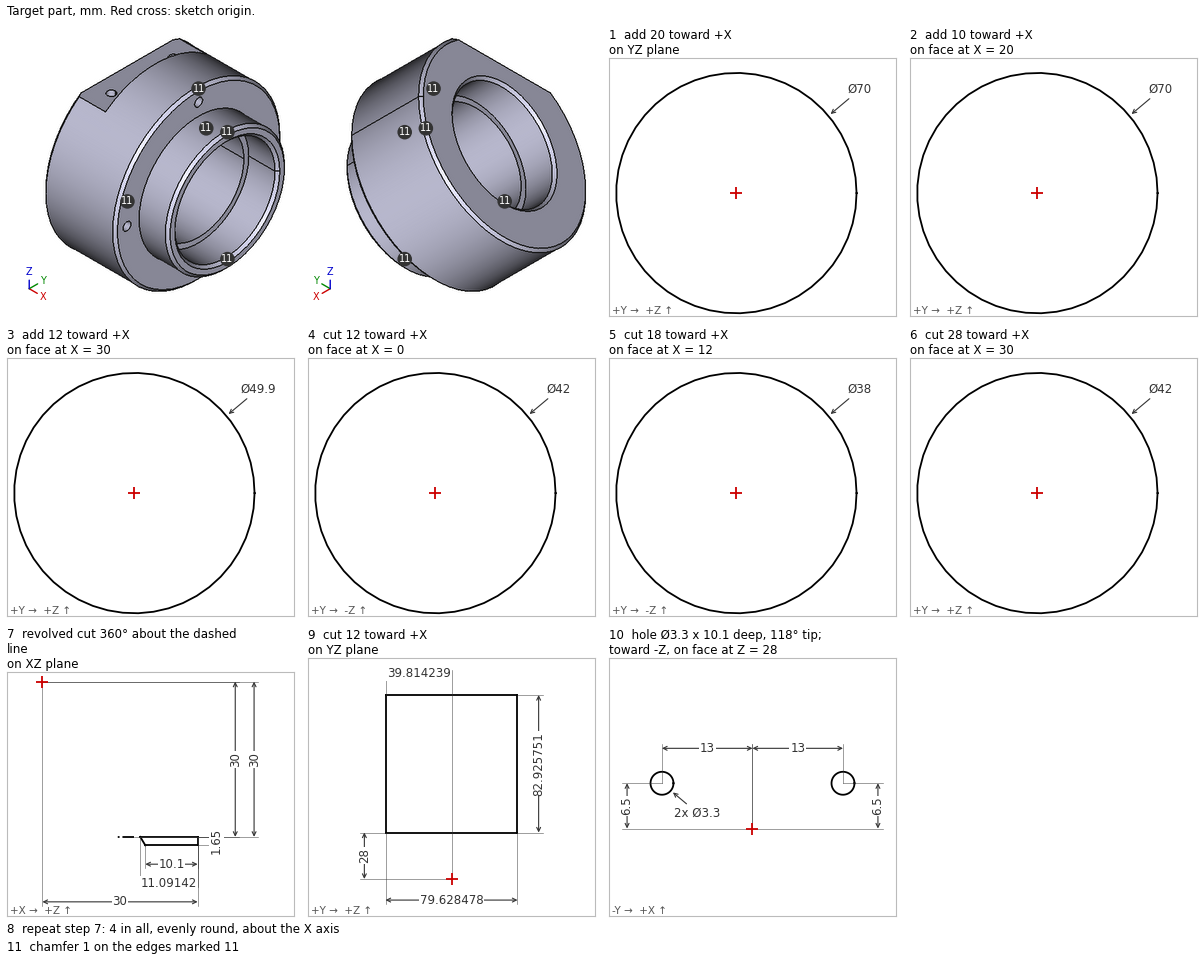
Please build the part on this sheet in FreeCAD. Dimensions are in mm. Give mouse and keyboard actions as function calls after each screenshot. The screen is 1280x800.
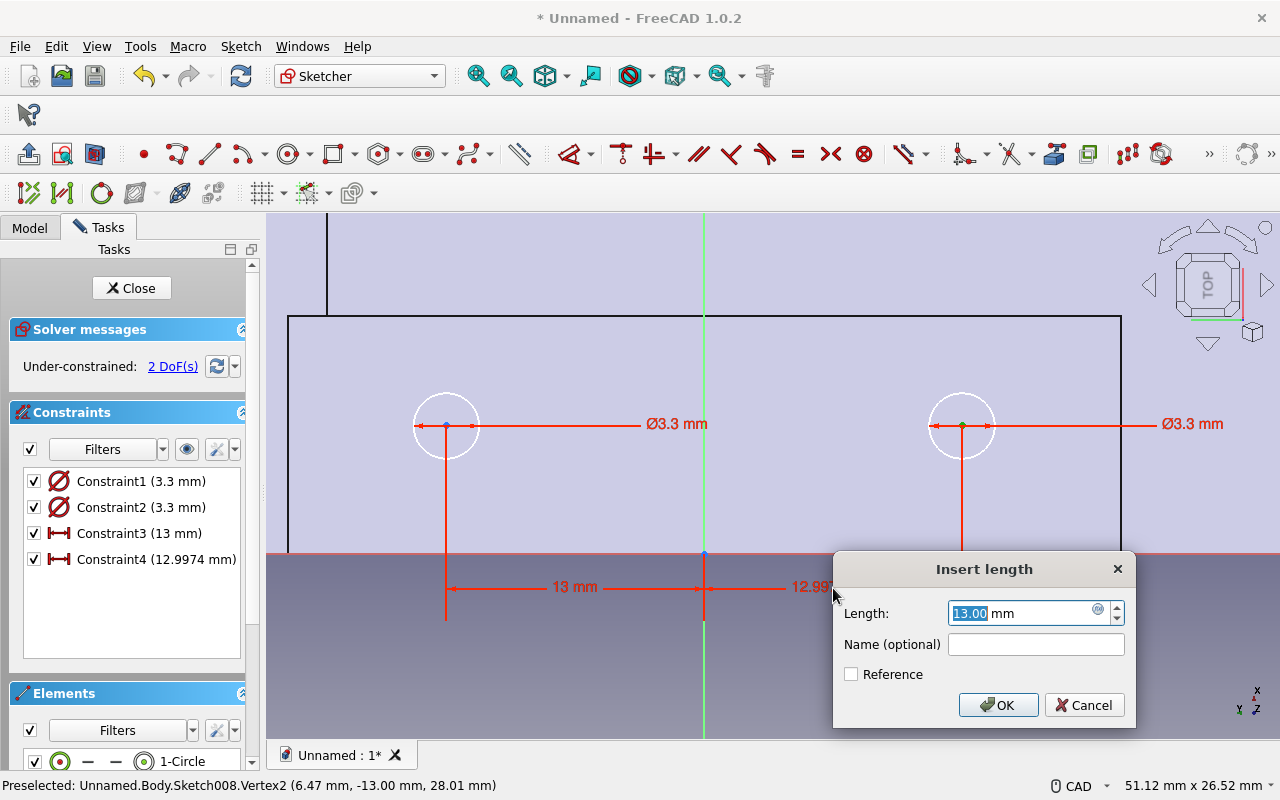
text(13)
key(Return)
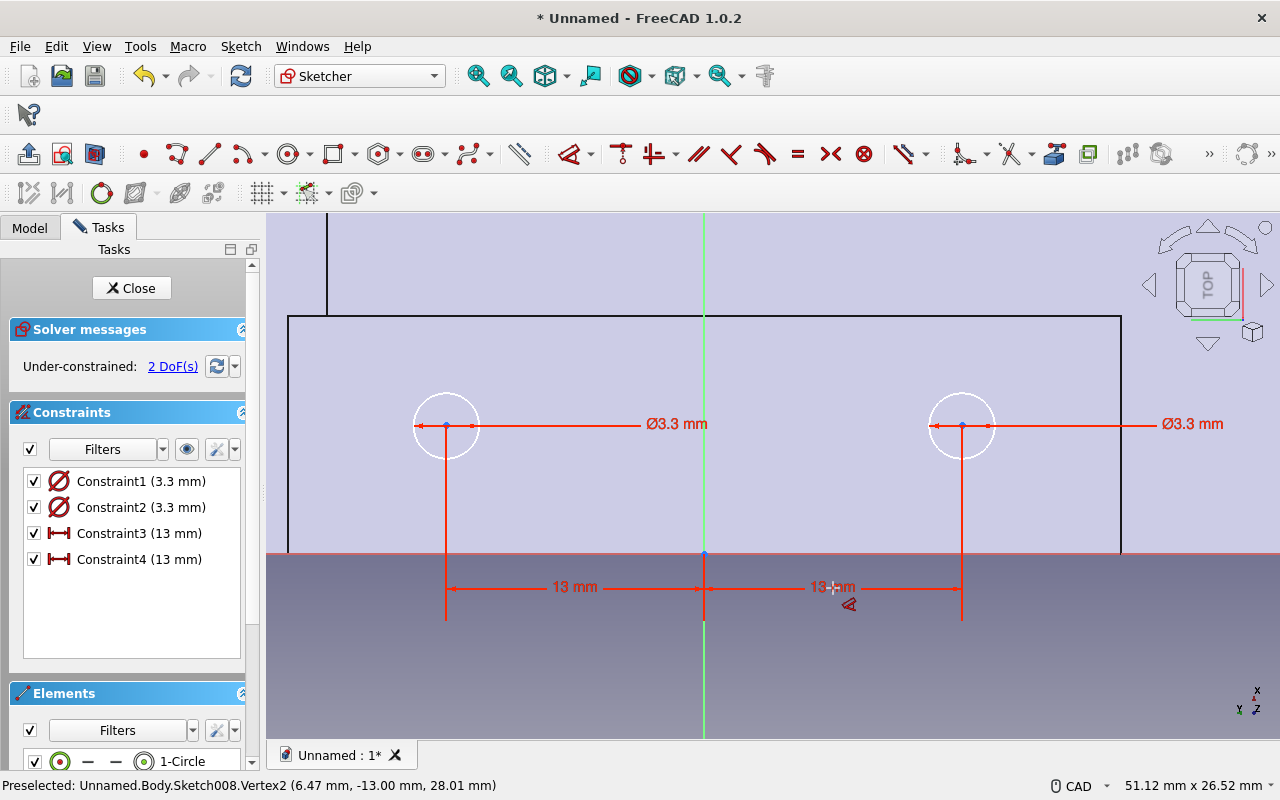
click(446, 426)
click(412, 490)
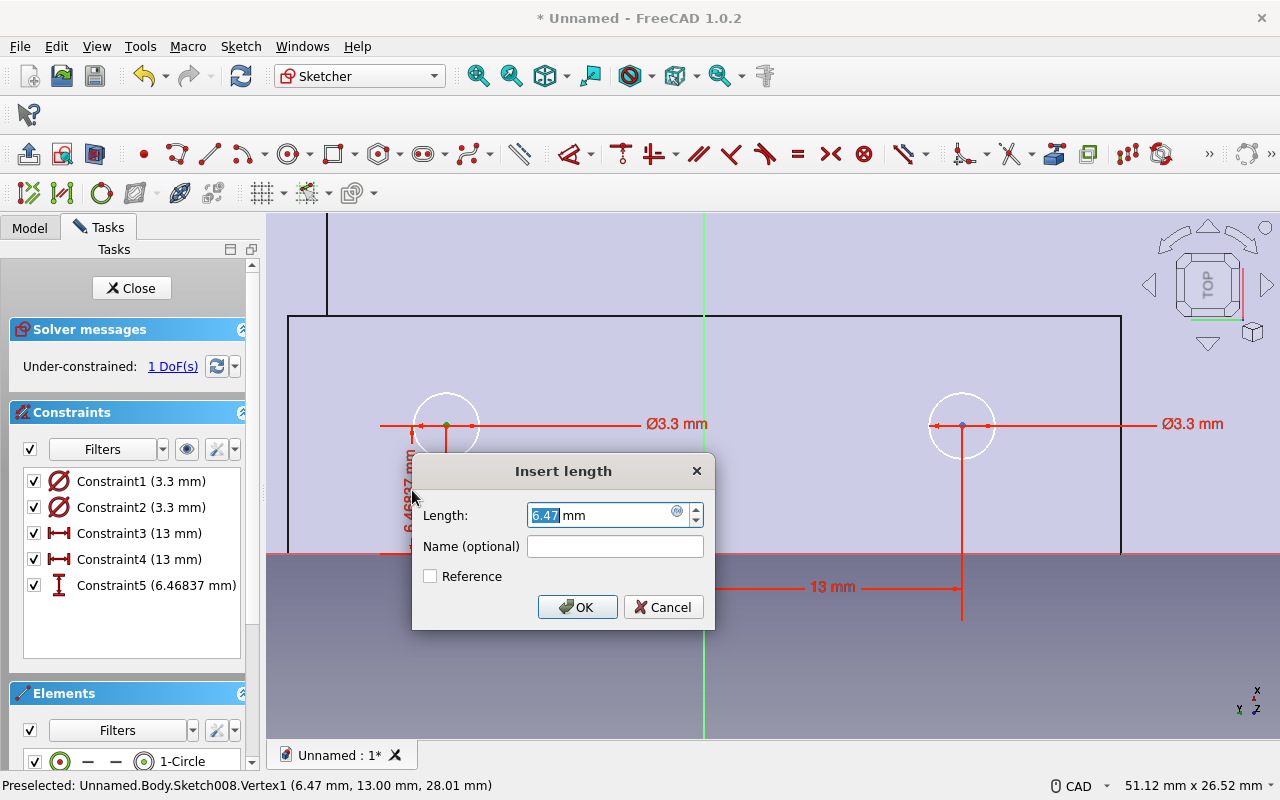
text(6.5)
key(Return)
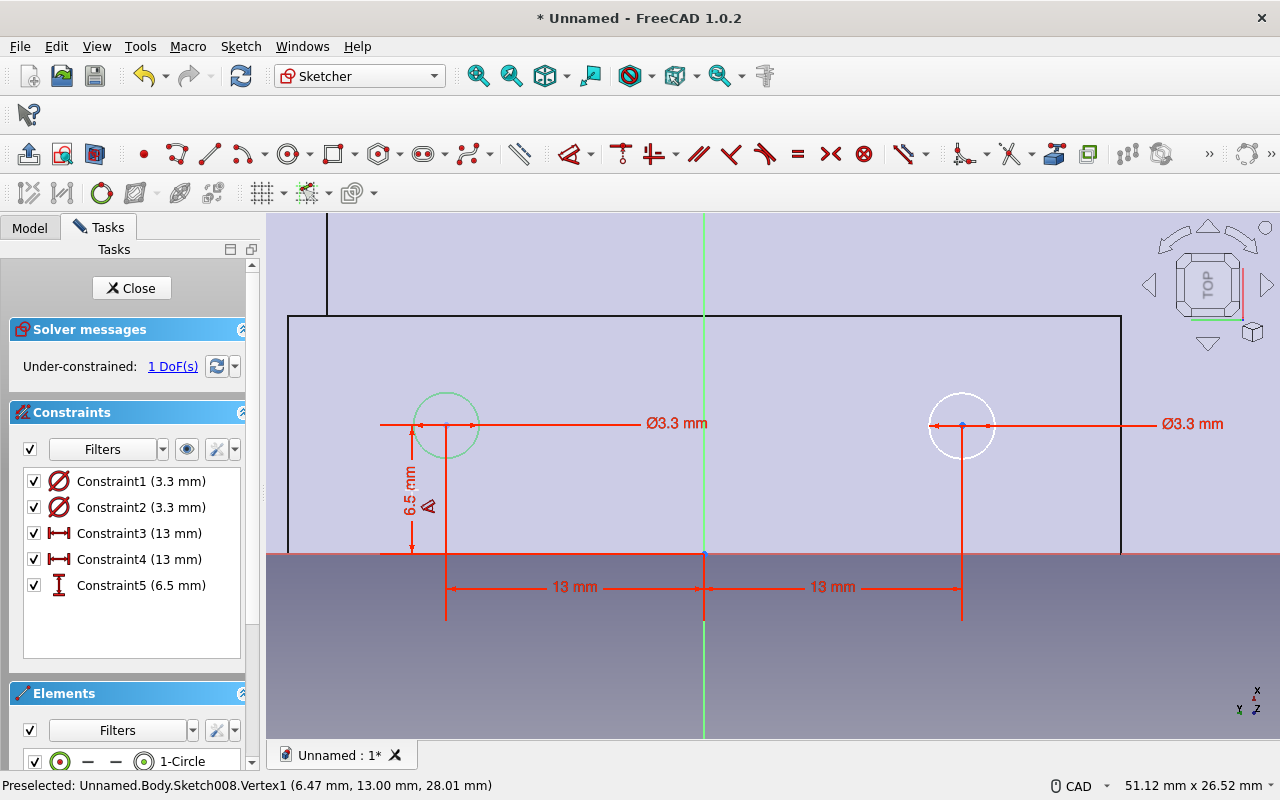
click(962, 426)
click(996, 490)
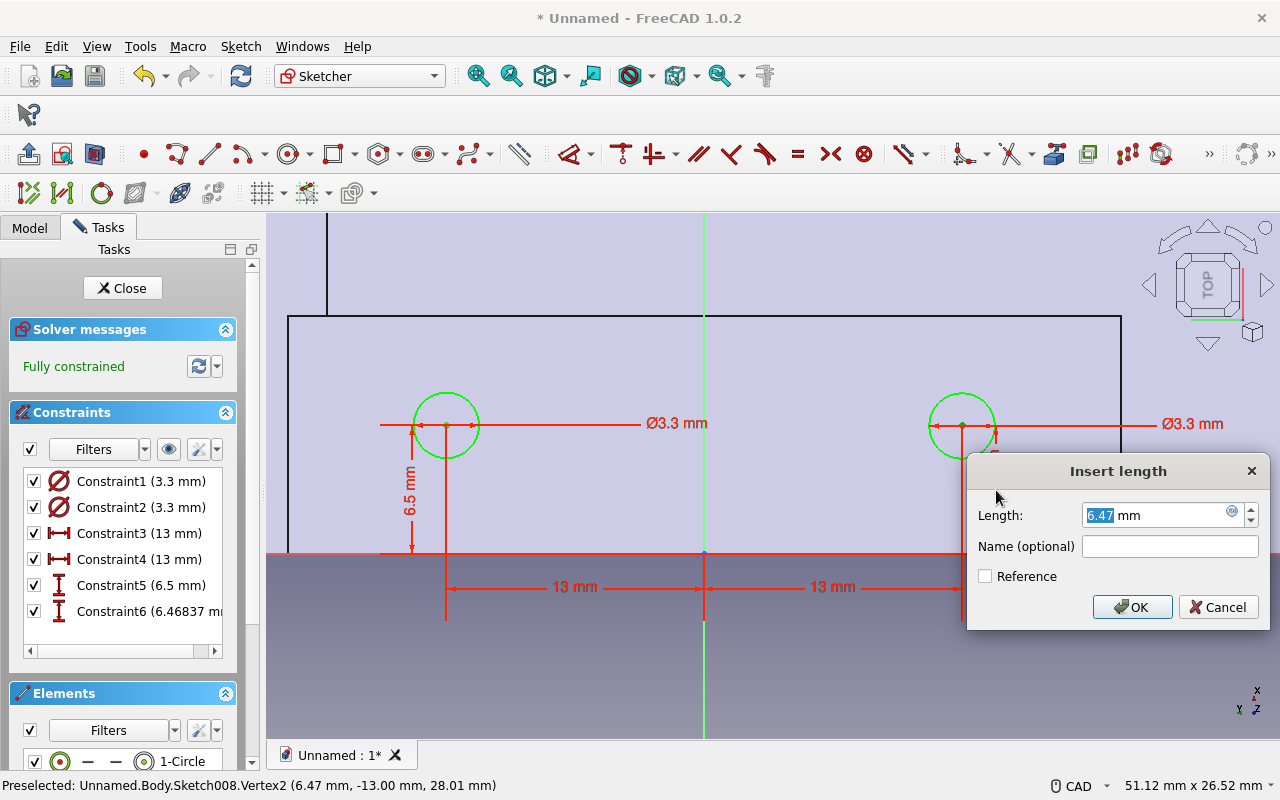
text(6.5)
key(Return)
key(Escape)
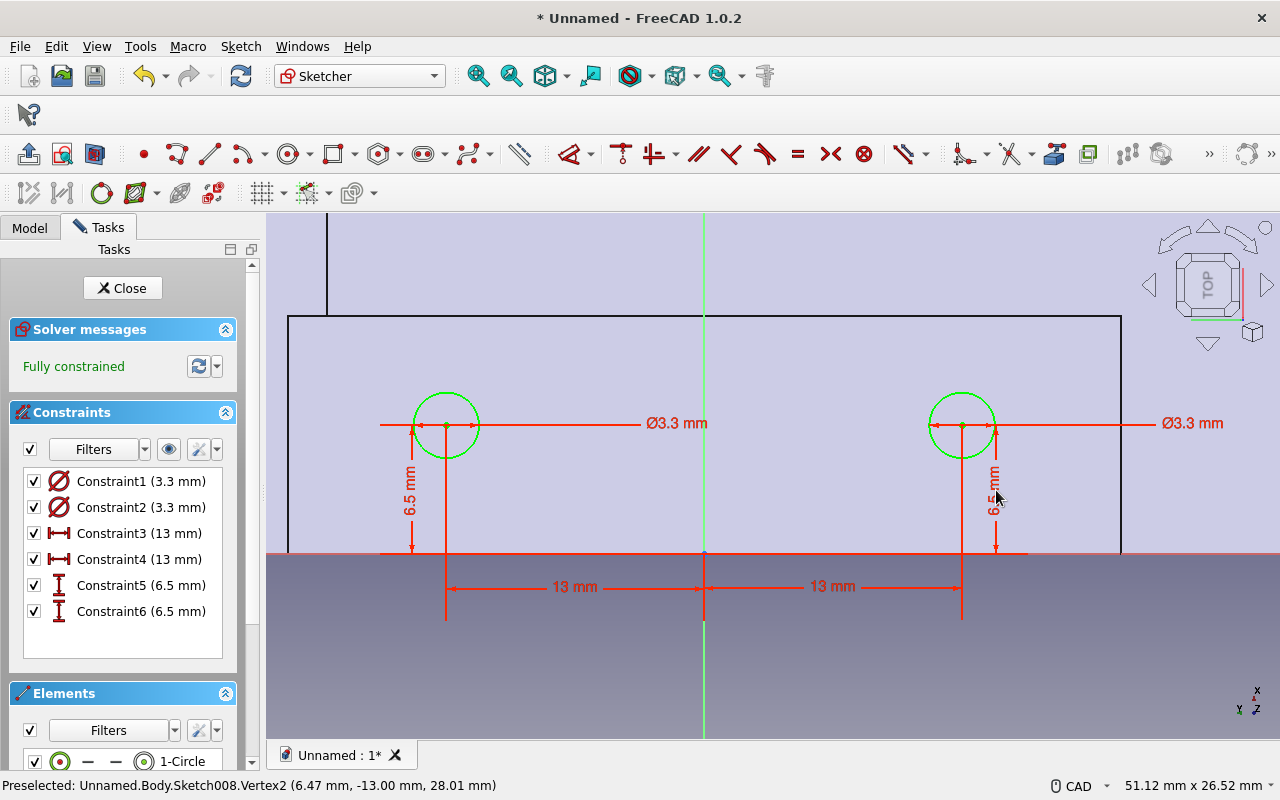
click(123, 288)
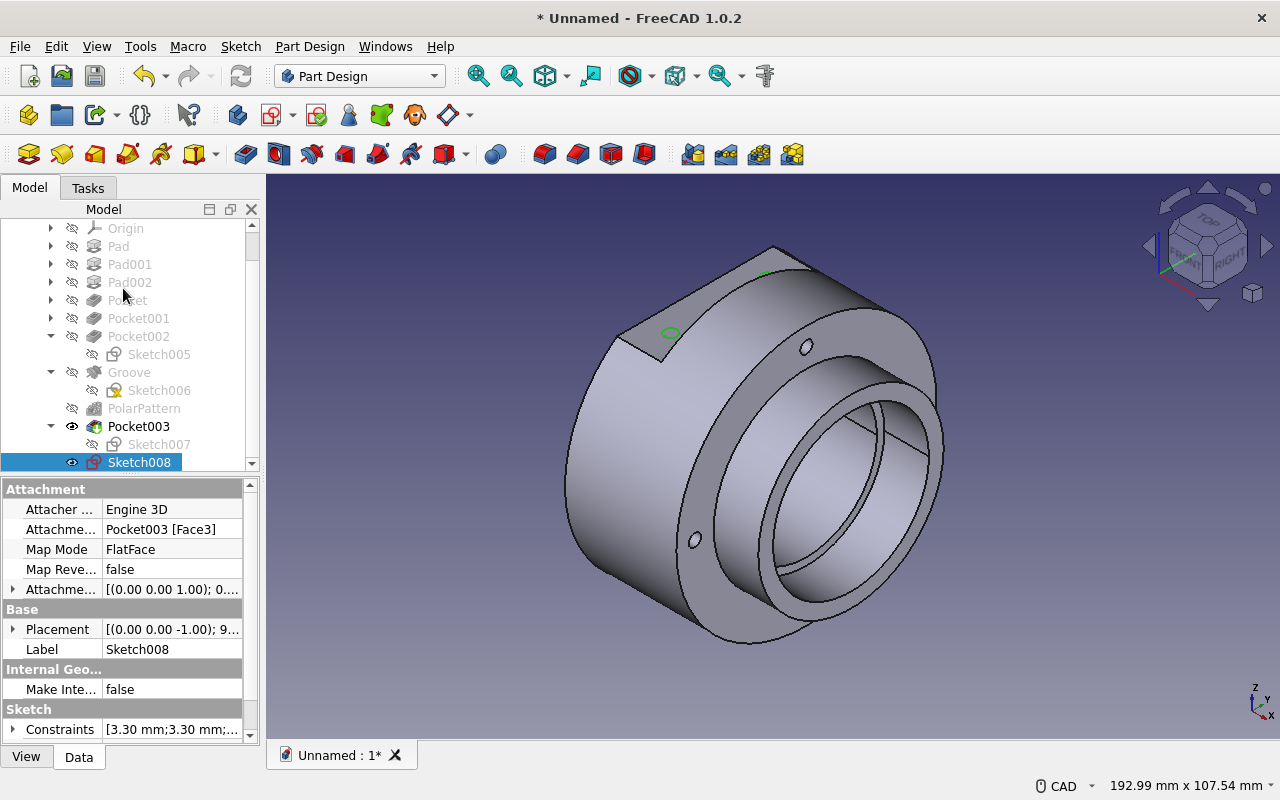
click(279, 154)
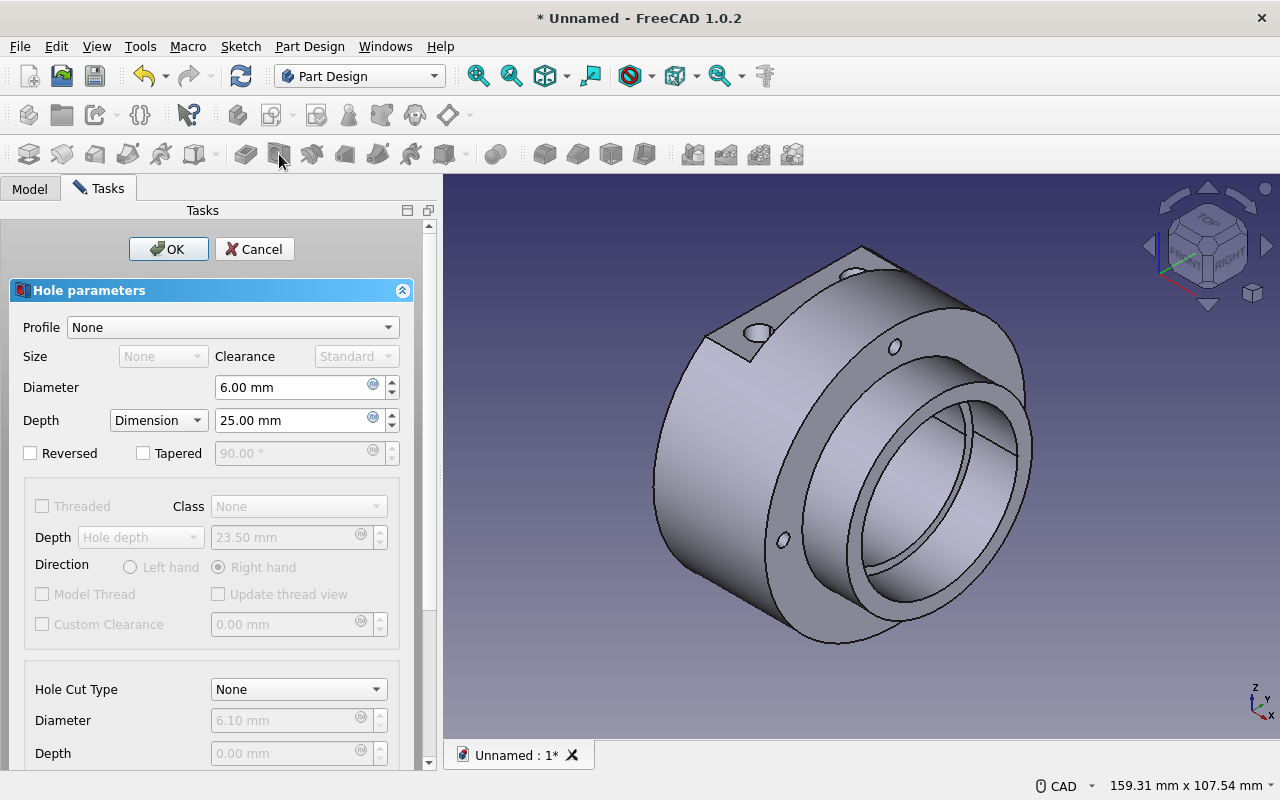
triple_click(300, 388)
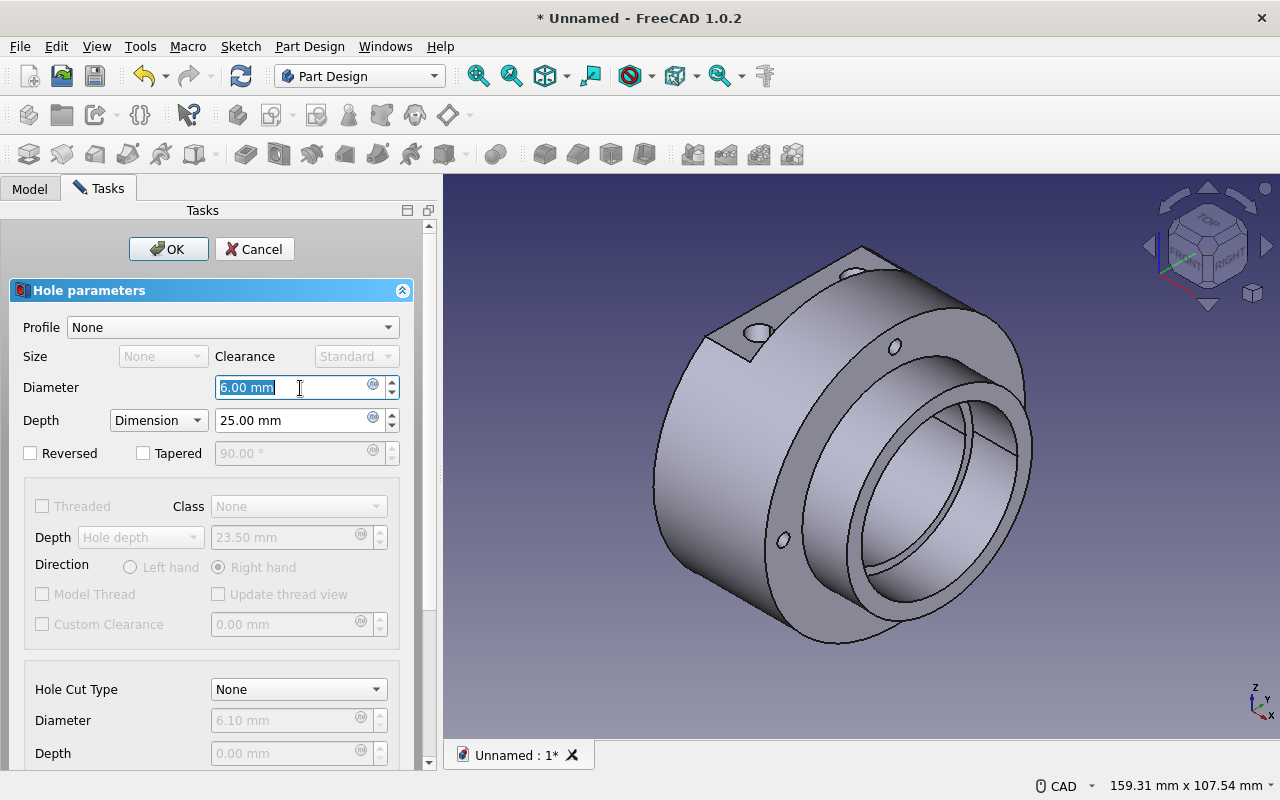
text(3.3)
key(Tab)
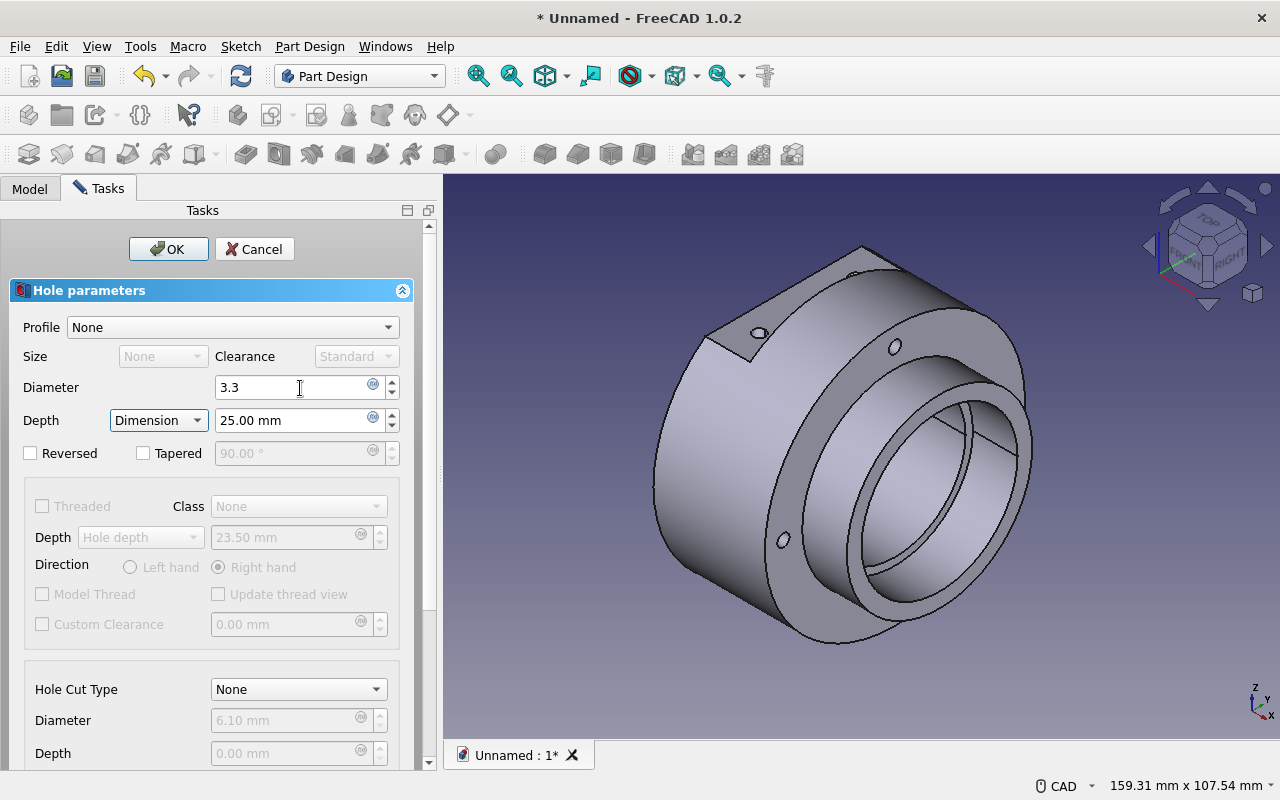
triple_click(300, 420)